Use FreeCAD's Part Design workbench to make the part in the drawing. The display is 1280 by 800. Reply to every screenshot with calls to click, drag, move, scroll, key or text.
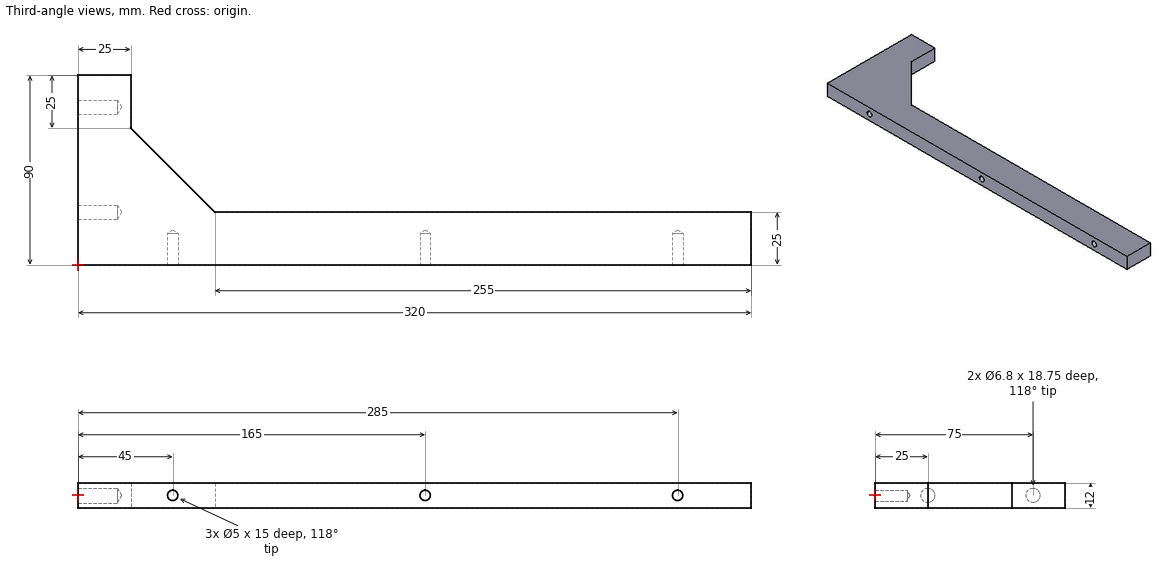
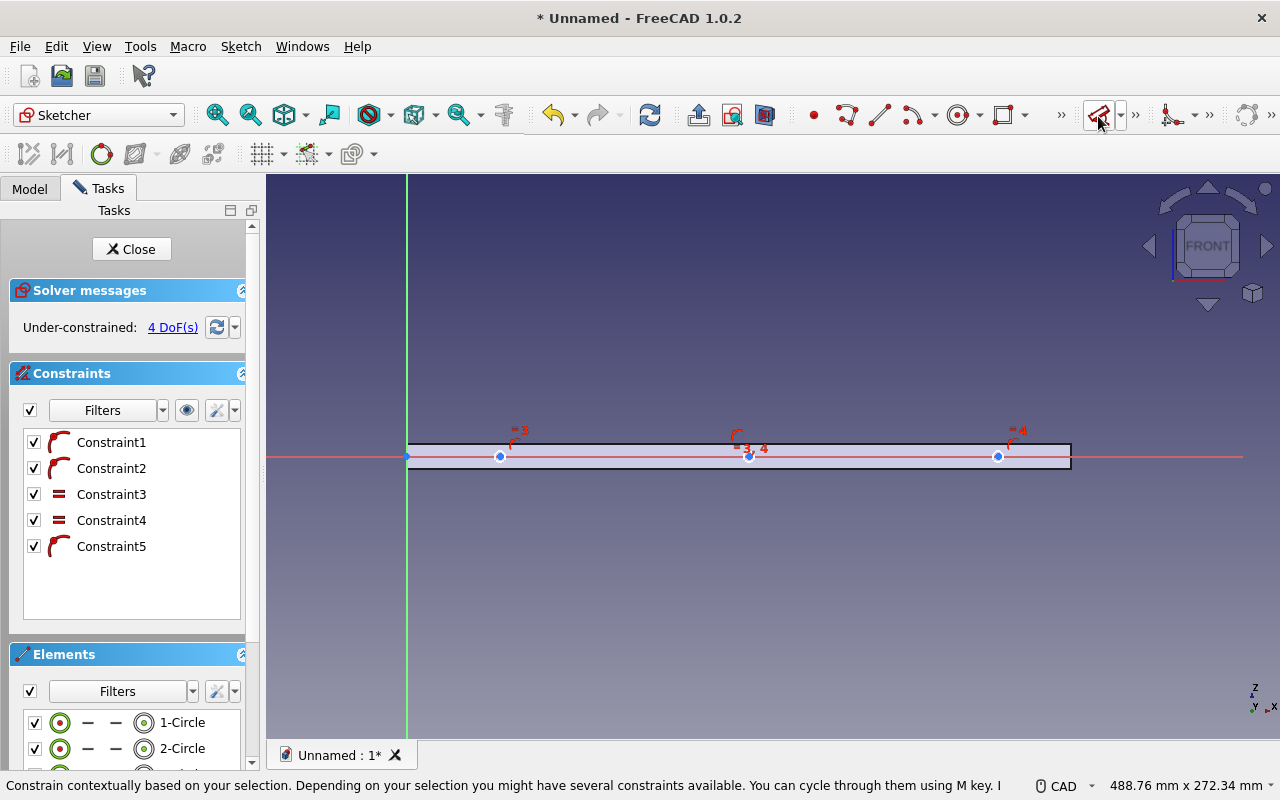
scroll(496, 460, up, 7)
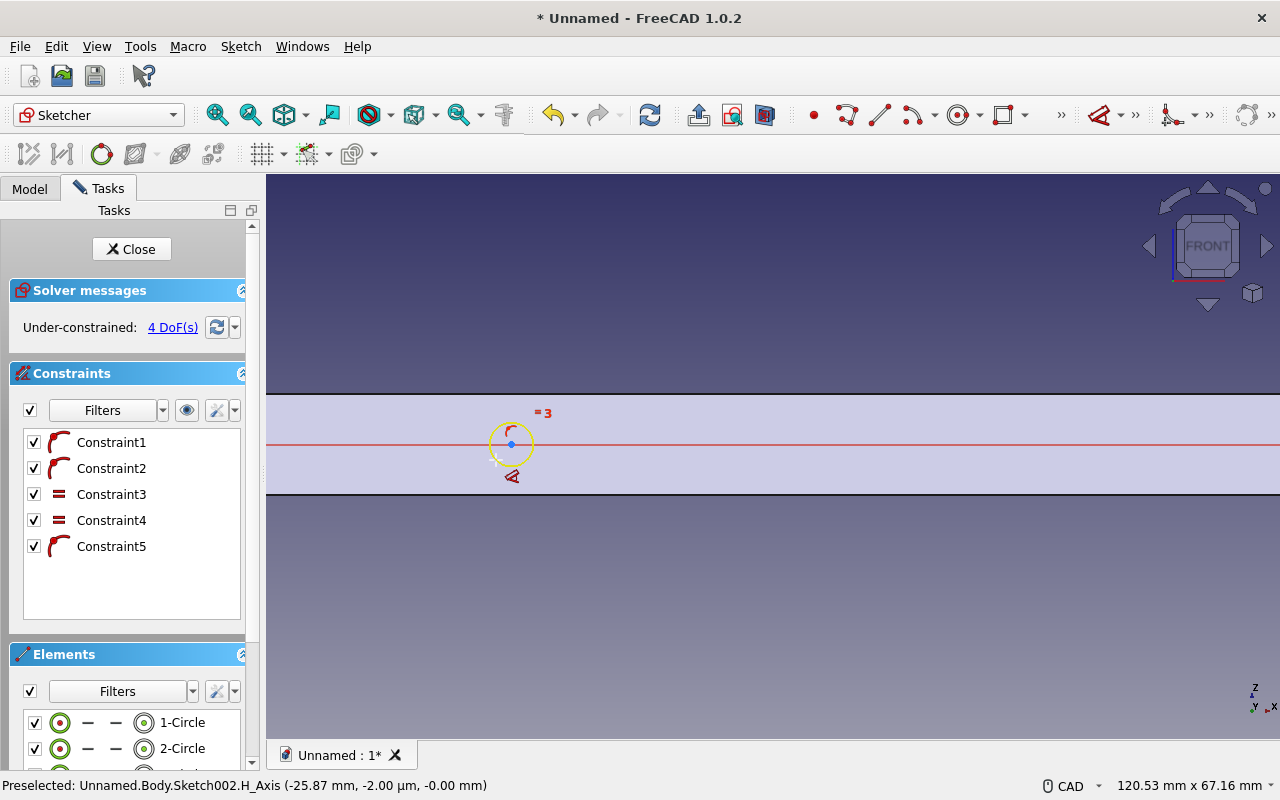
click(496, 460)
click(473, 482)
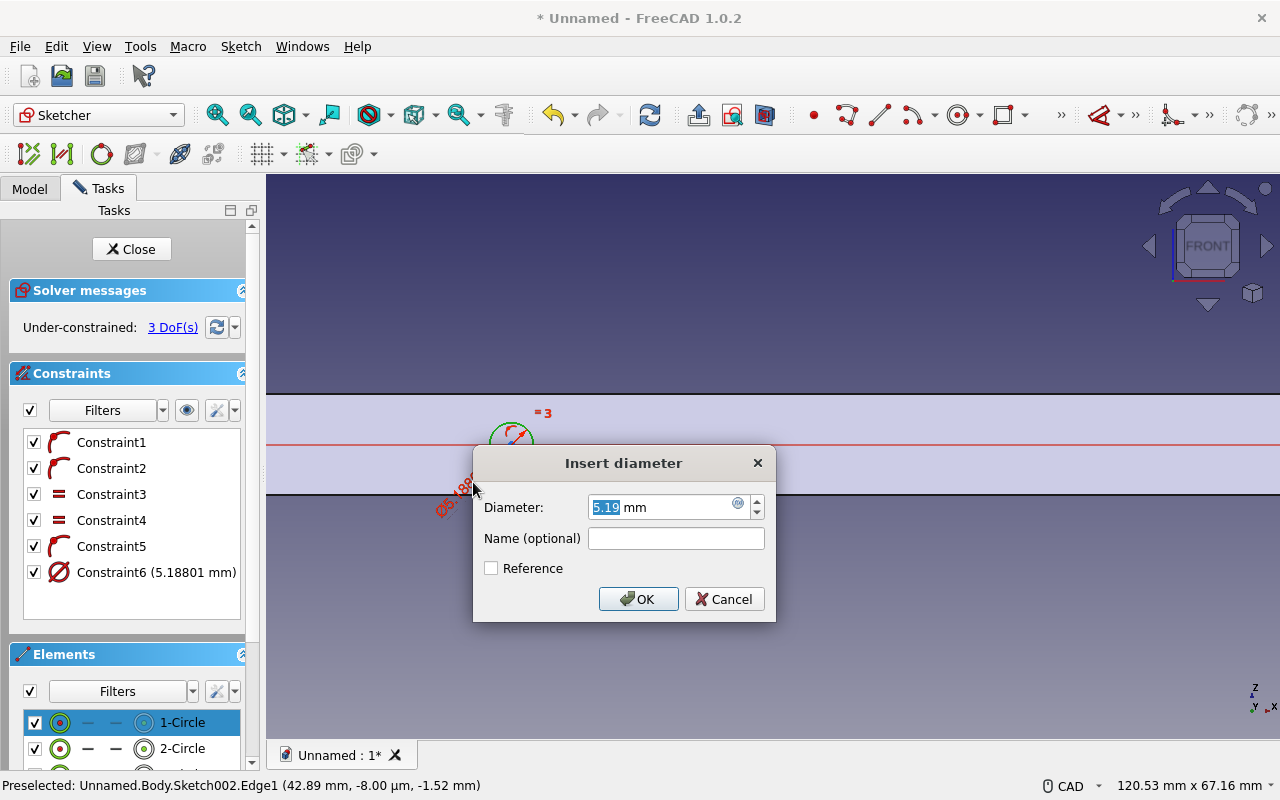
text(5)
key(Return)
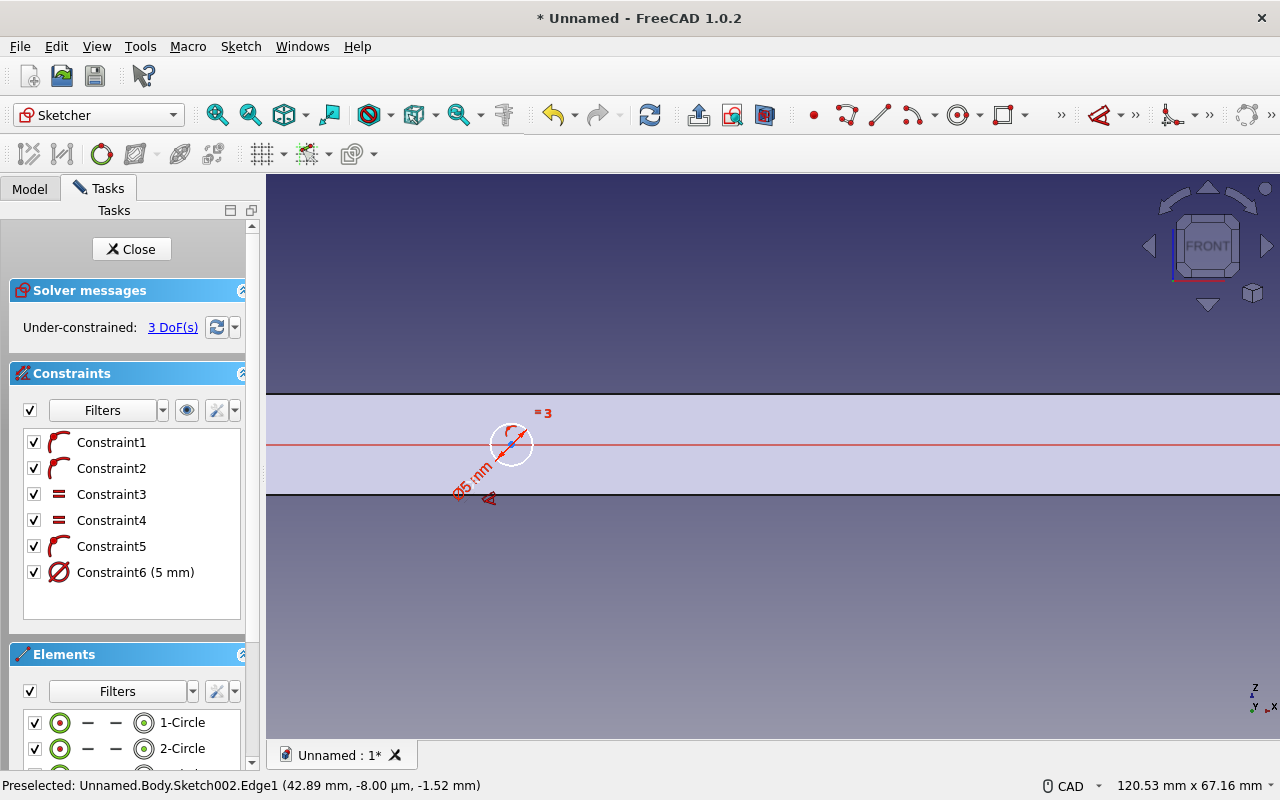
scroll(496, 460, down, 7)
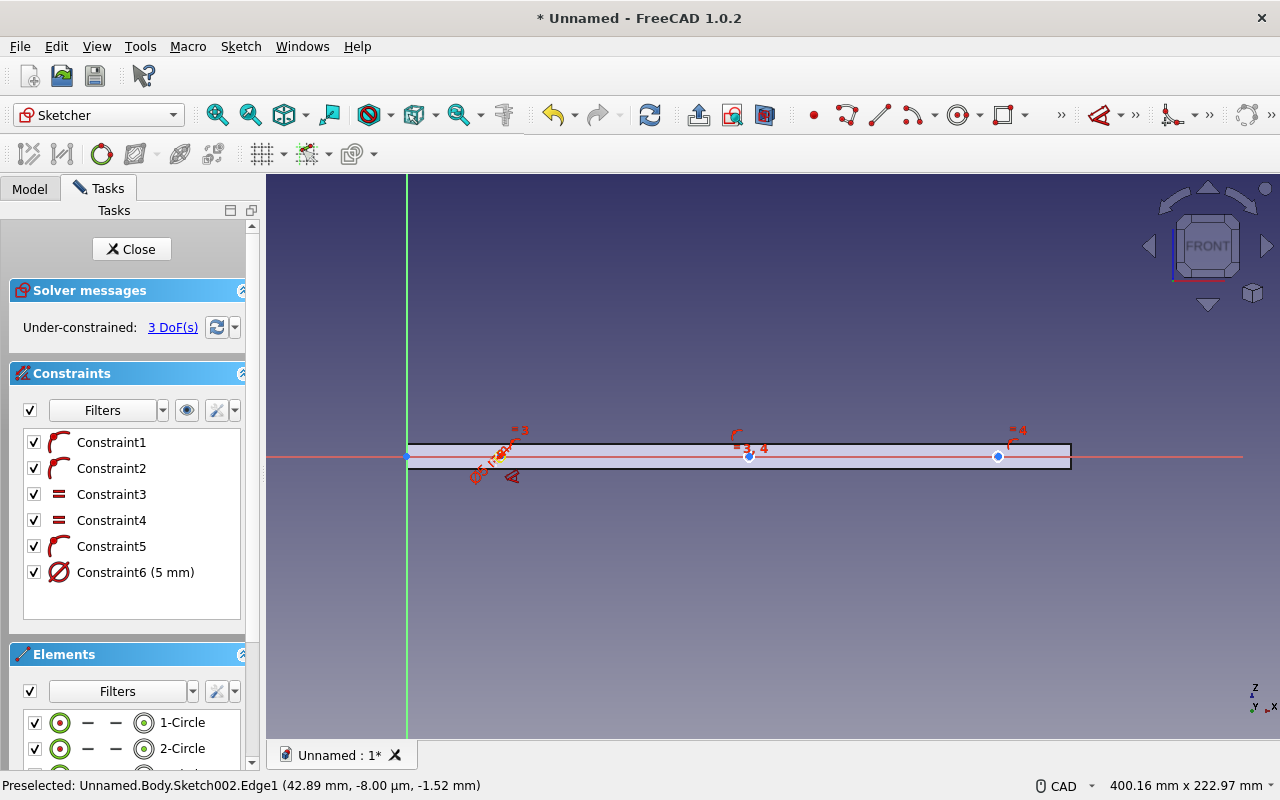
click(500, 457)
click(453, 491)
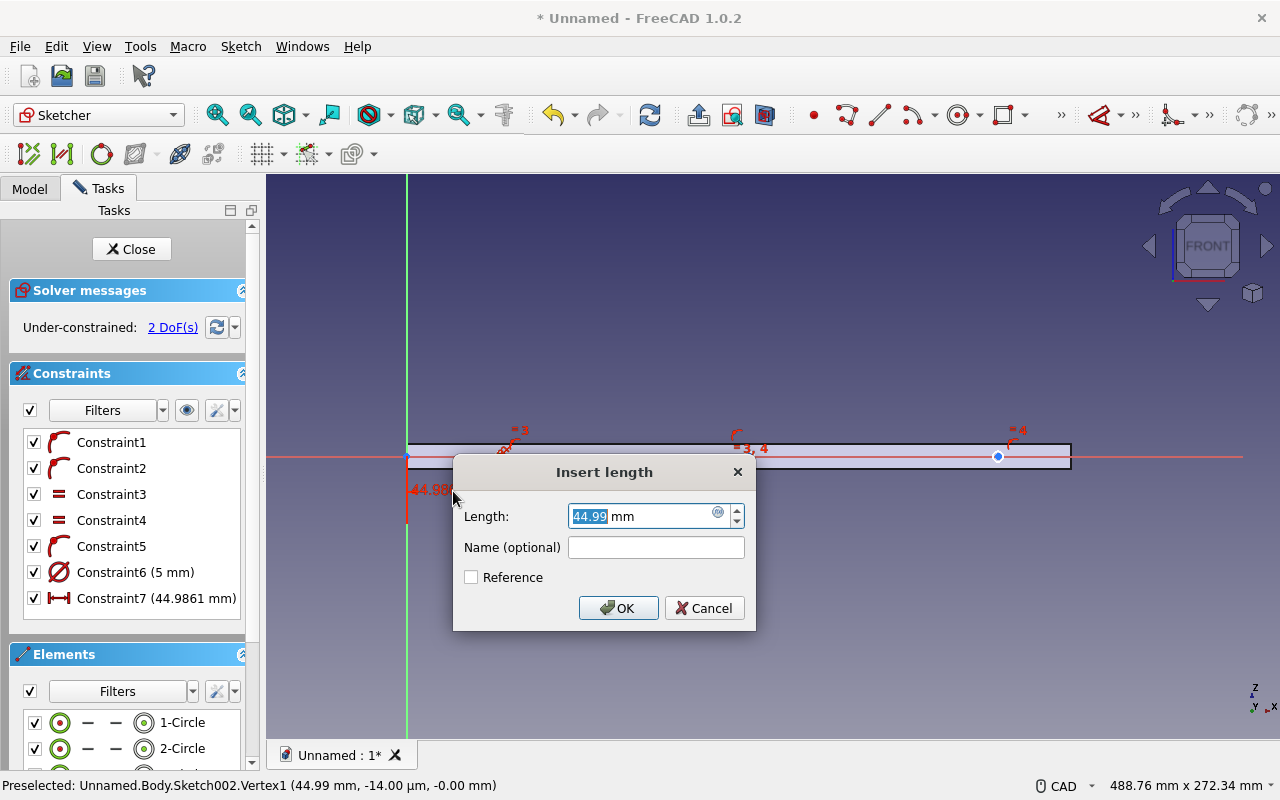
text(45)
key(Return)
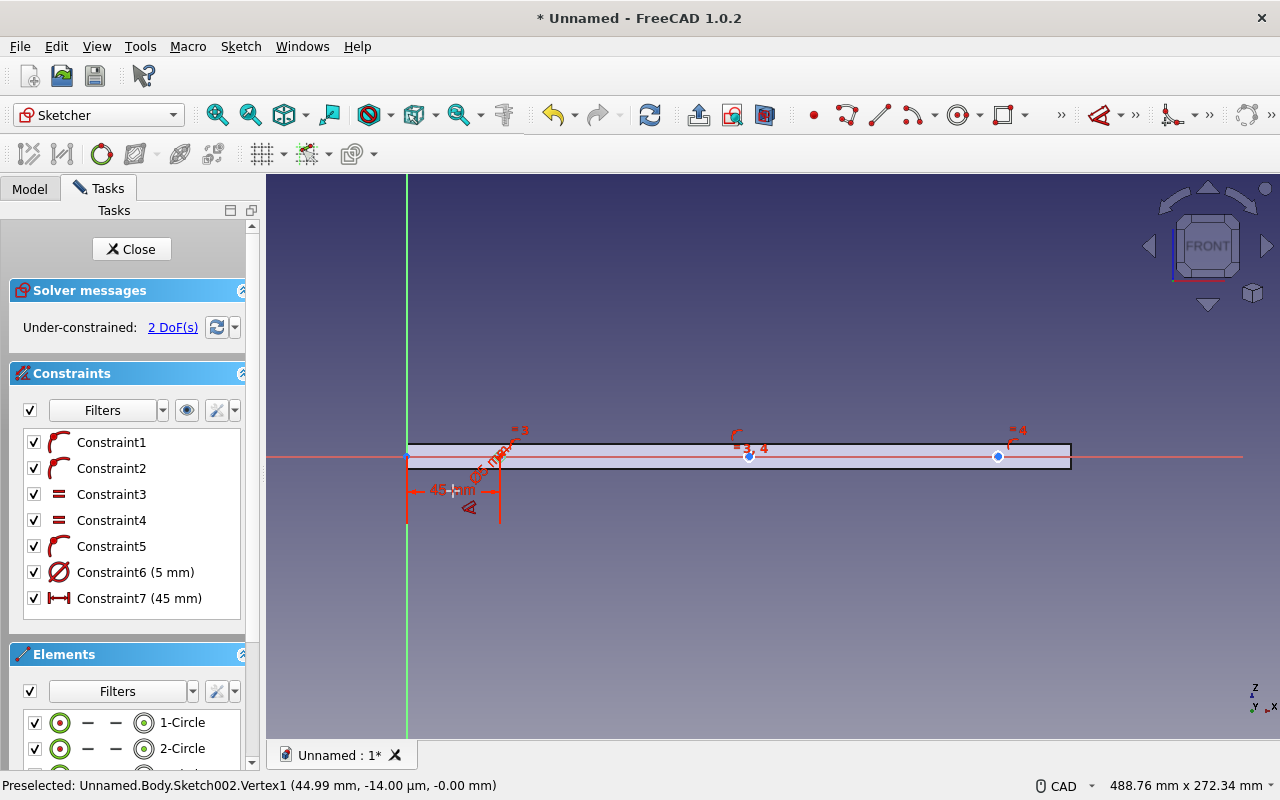
click(749, 457)
click(578, 491)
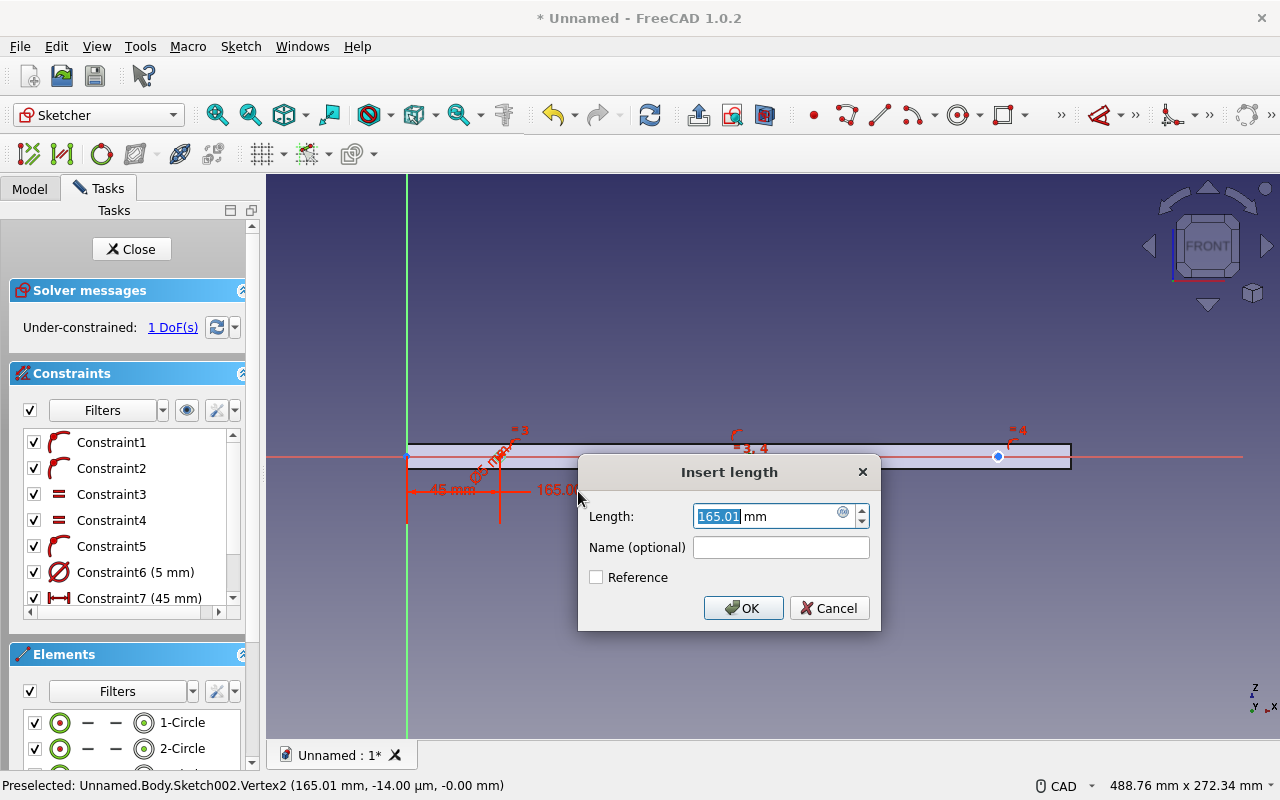
text(165)
key(Return)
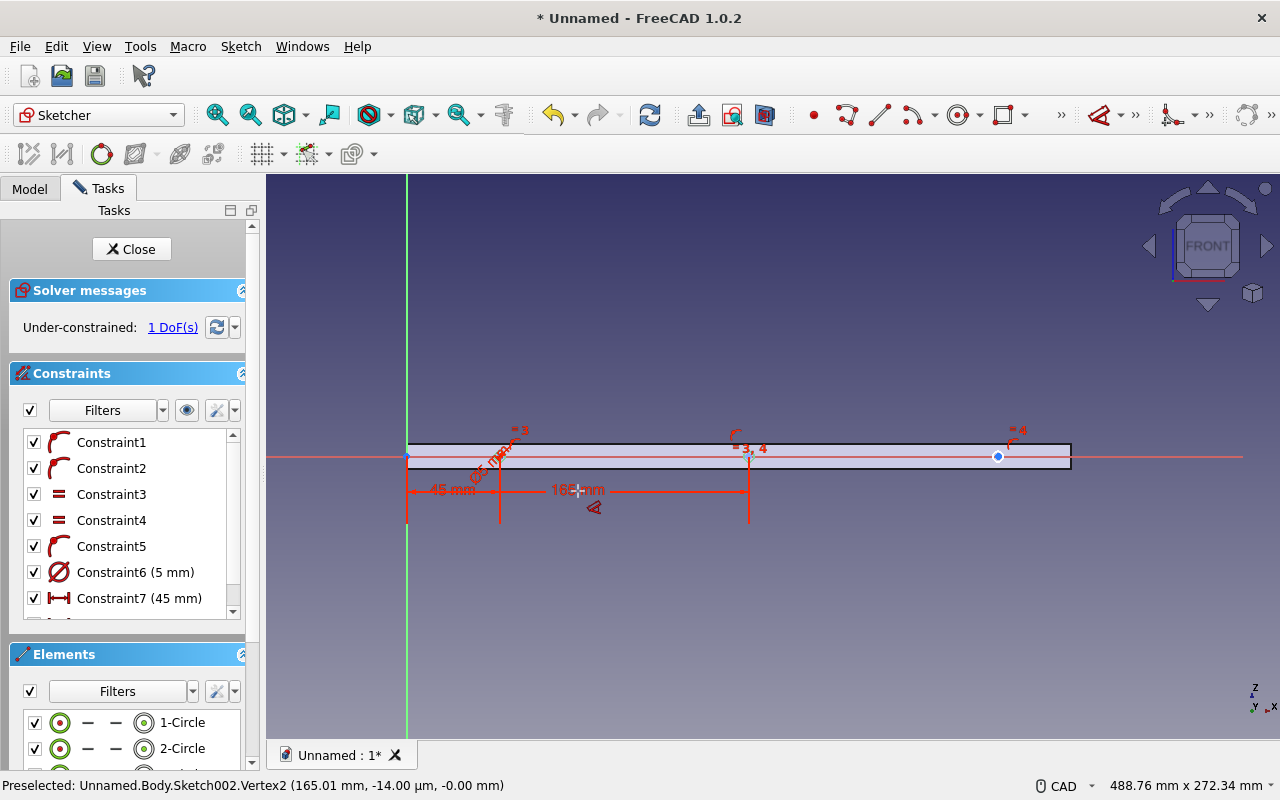
click(998, 457)
click(702, 491)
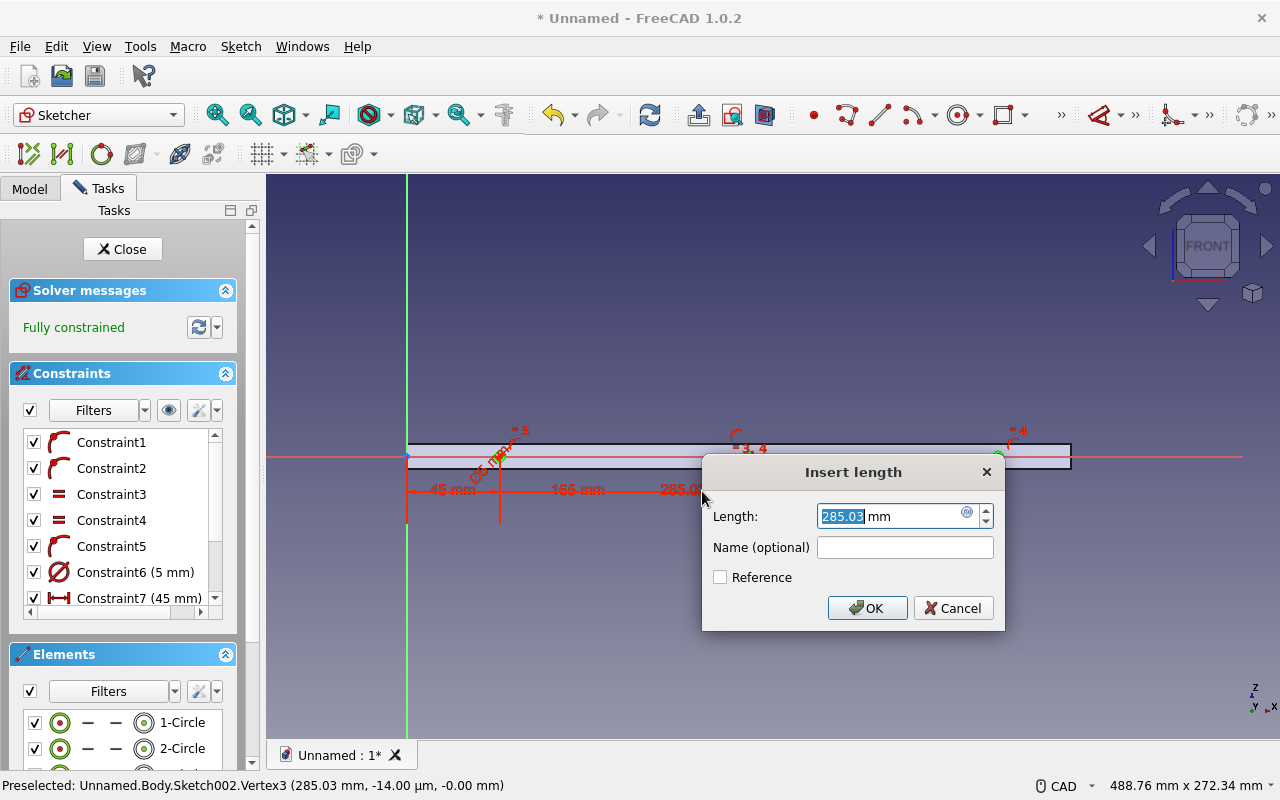
text(285)
key(Return)
key(Escape)